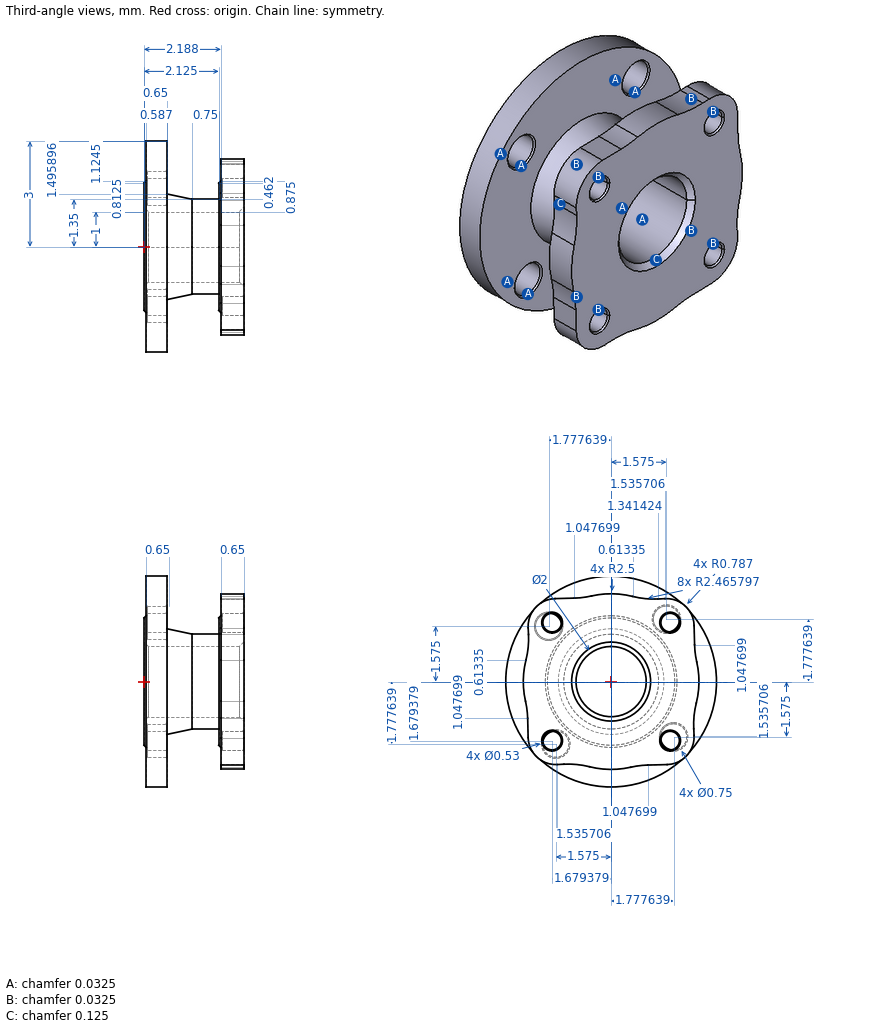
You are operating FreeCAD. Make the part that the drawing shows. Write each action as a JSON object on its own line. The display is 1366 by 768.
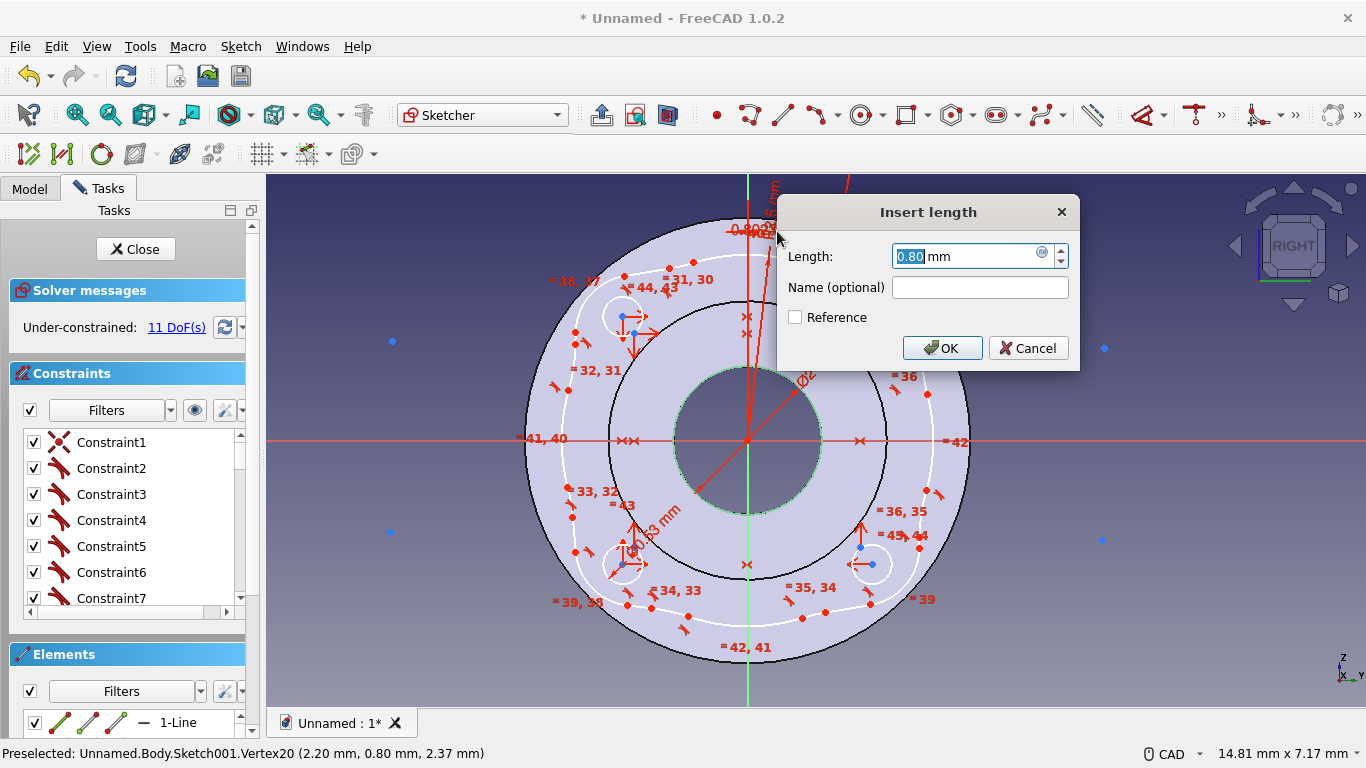
{"action": "type", "text": "0.61335"}
{"action": "key", "text": "Return"}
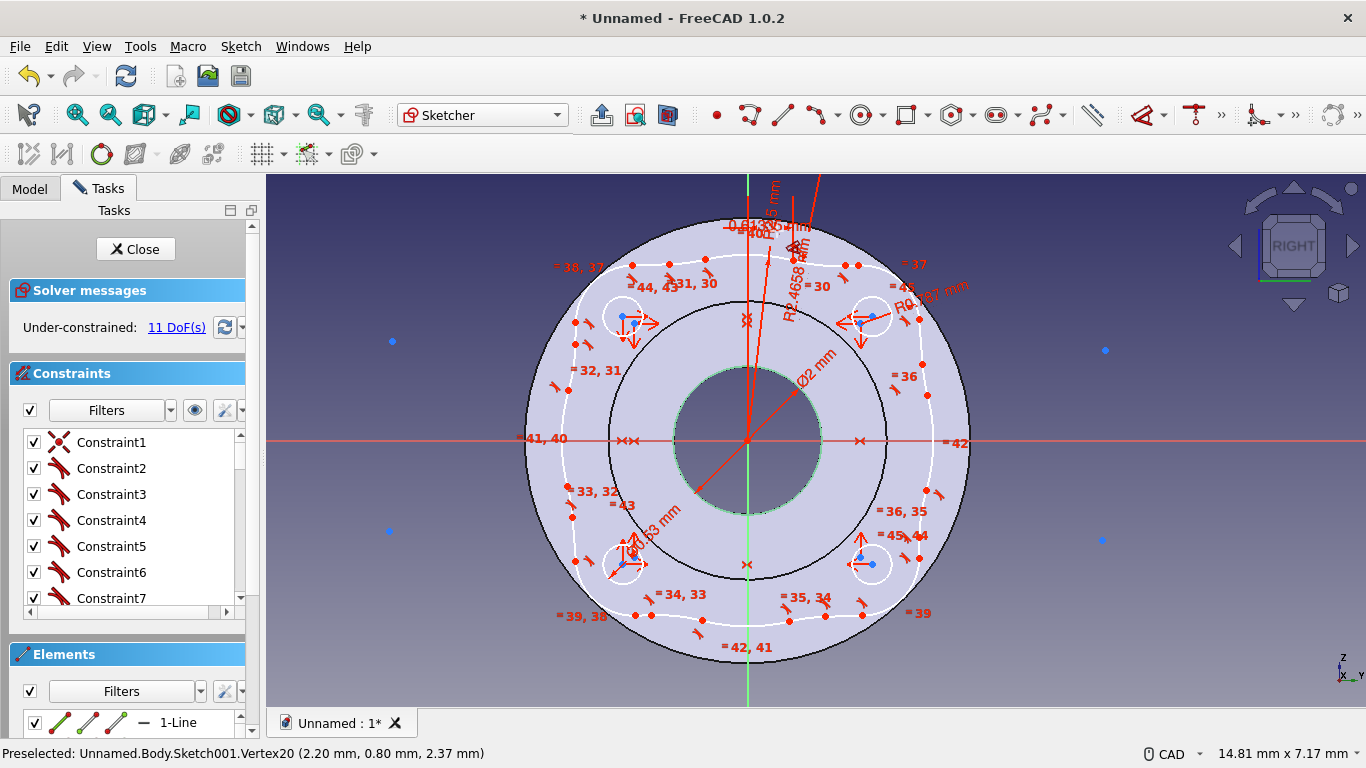
{"action": "left_click", "coordinate": [569, 391]}
{"action": "left_click", "coordinate": [535, 416]}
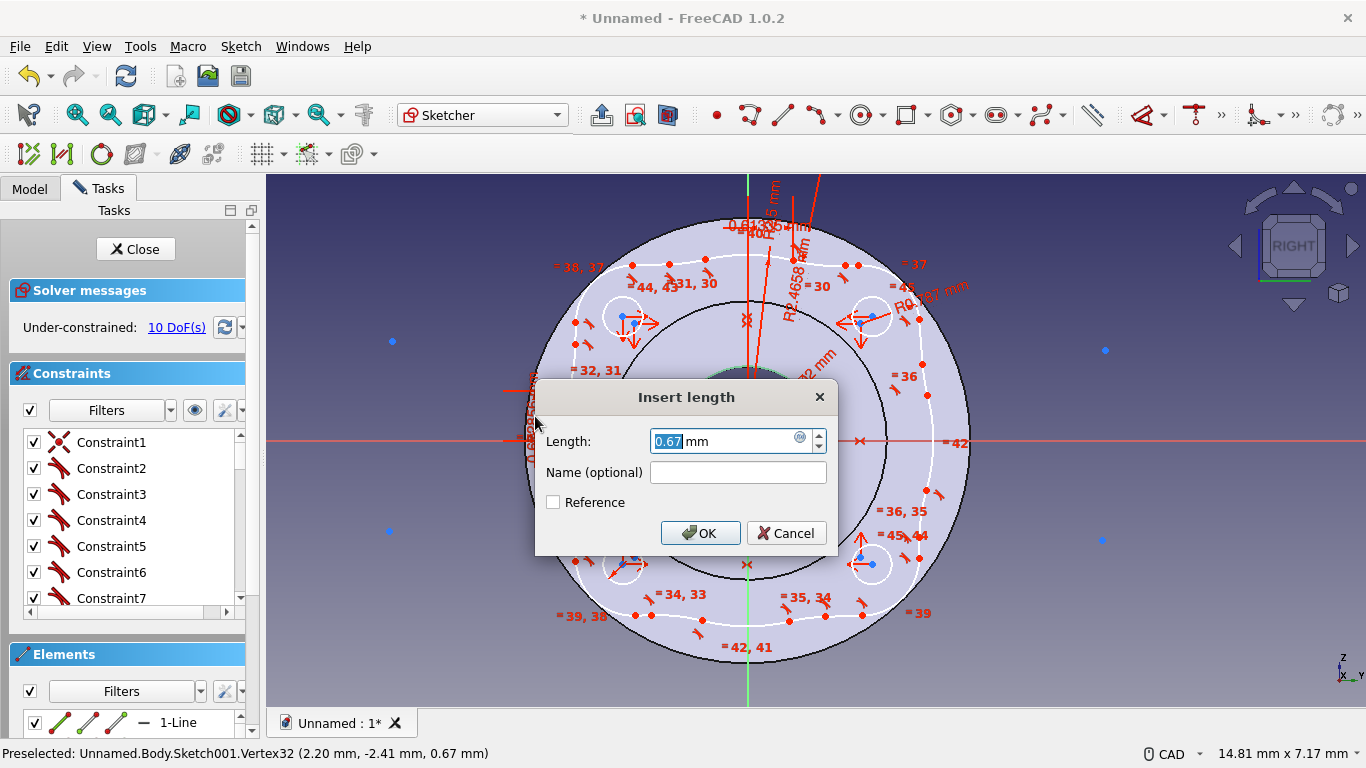
{"action": "type", "text": "0.61335"}
{"action": "key", "text": "Return"}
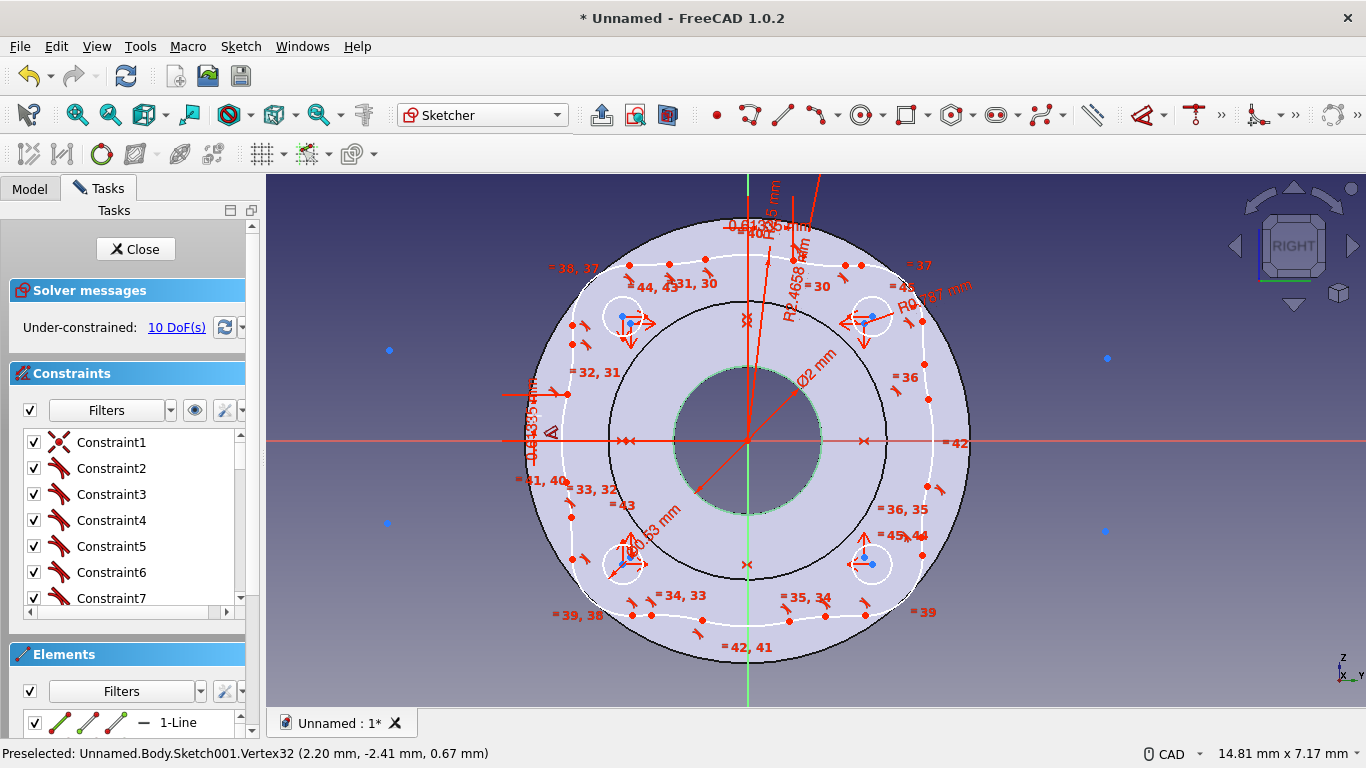
{"action": "left_click", "coordinate": [623, 564]}
{"action": "left_click", "coordinate": [685, 598]}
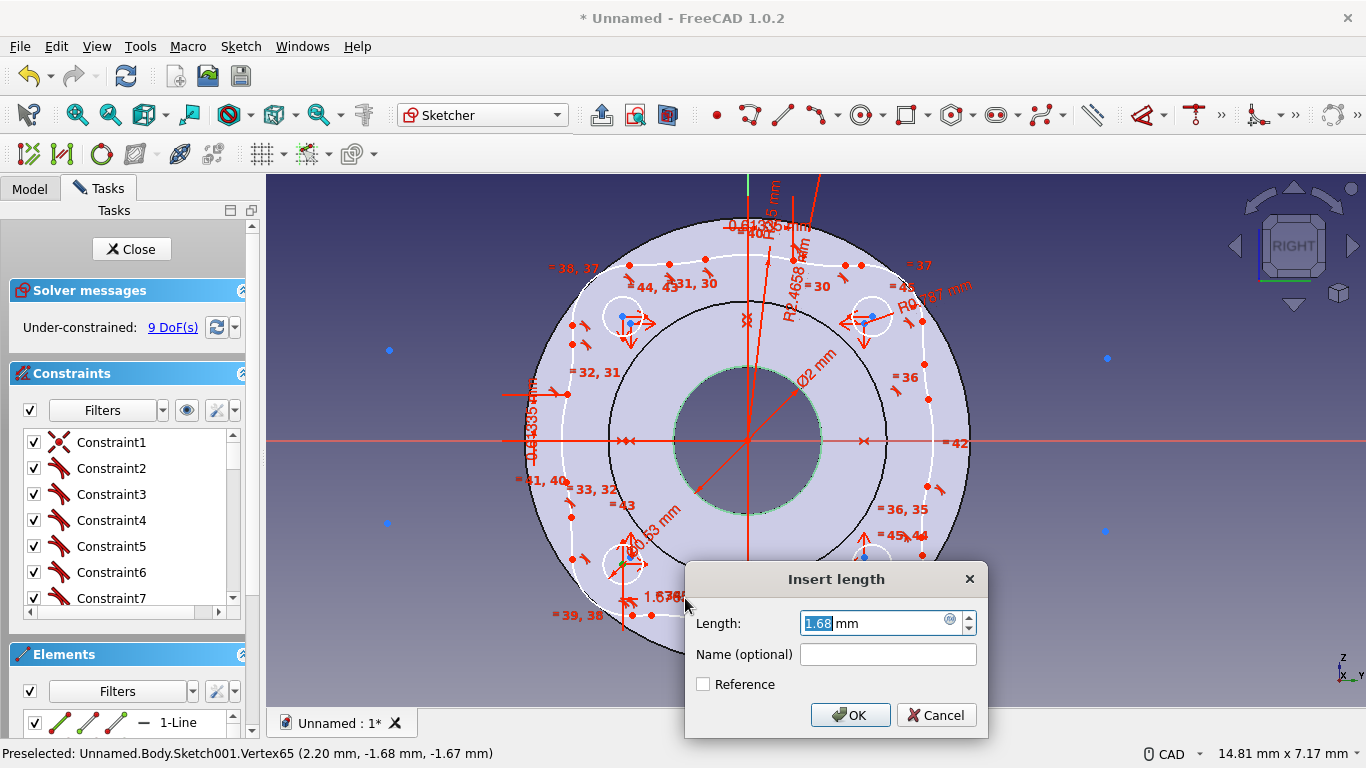
{"action": "type", "text": "1.679379"}
{"action": "key", "text": "Return"}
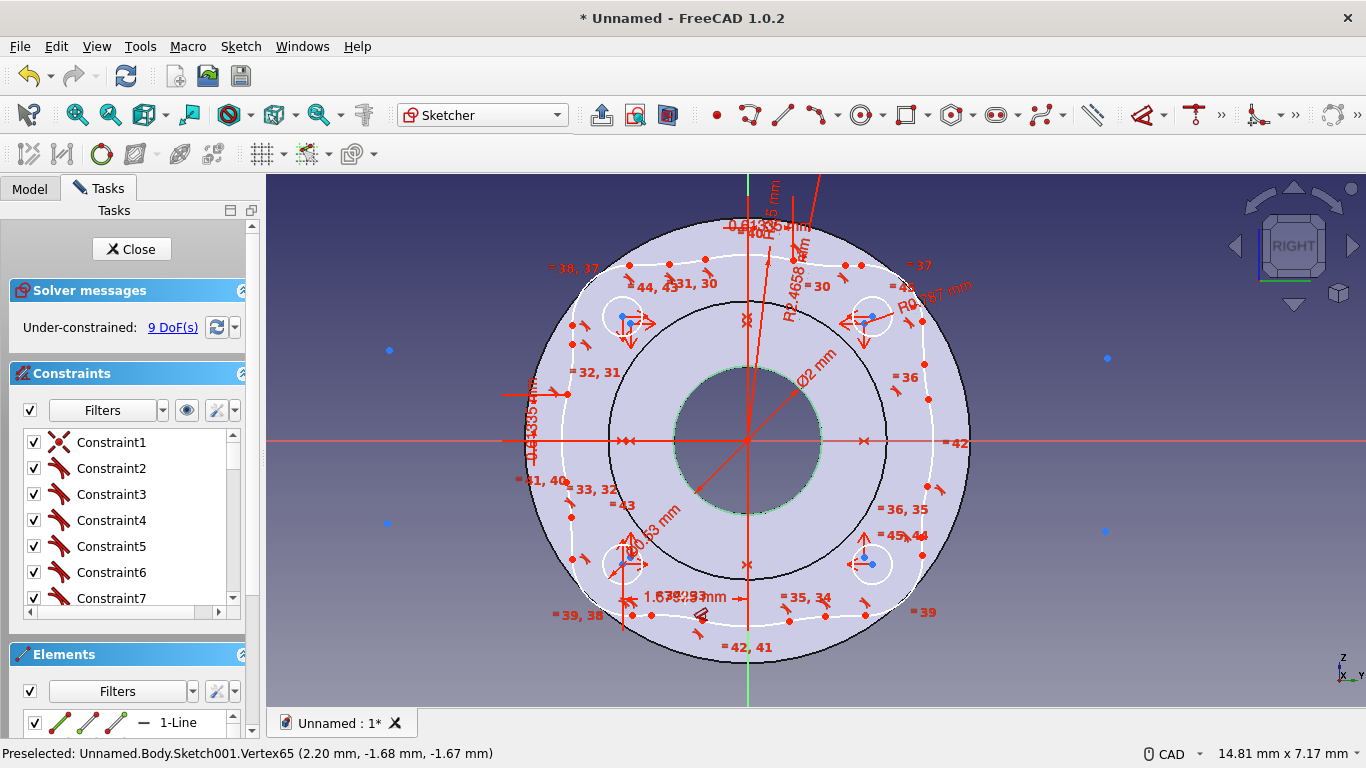
{"action": "left_click", "coordinate": [623, 564]}
{"action": "left_click", "coordinate": [589, 503]}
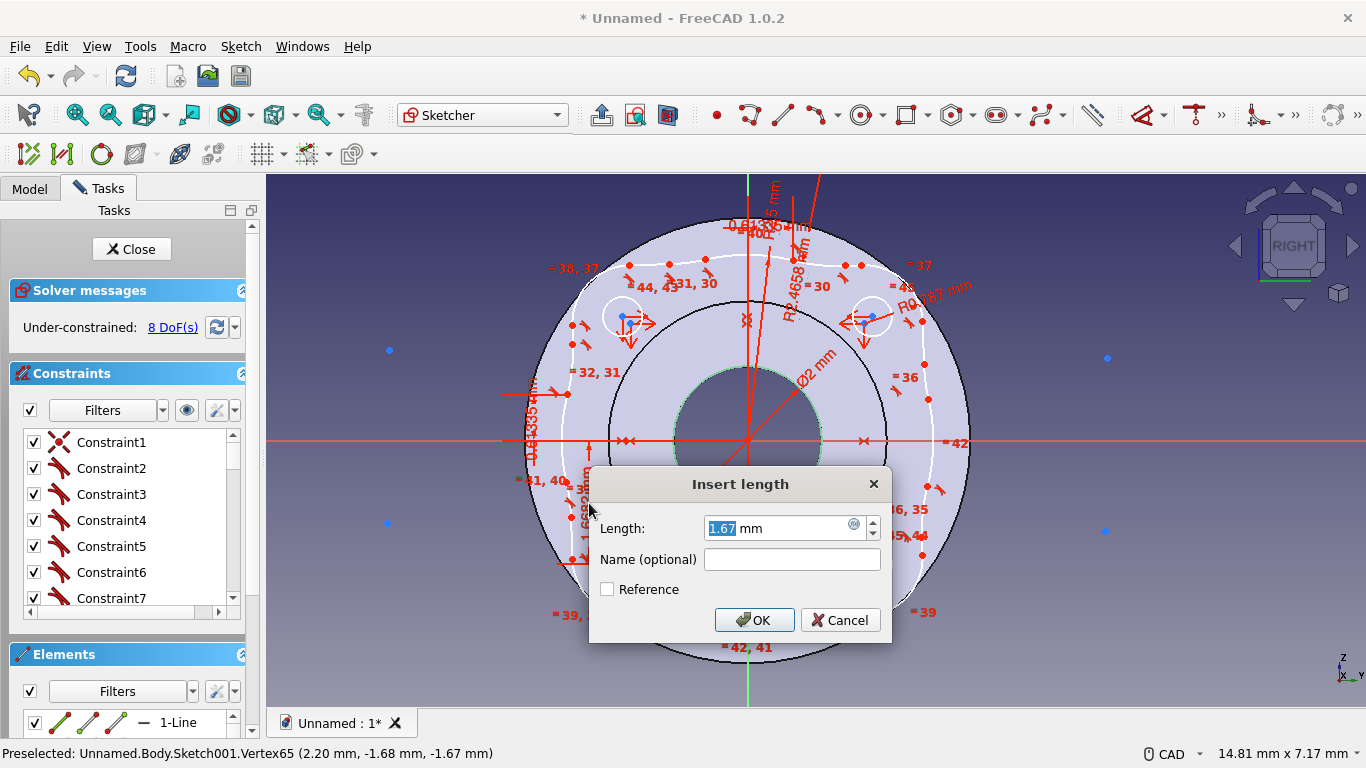
{"action": "type", "text": "1.679379"}
{"action": "key", "text": "Return"}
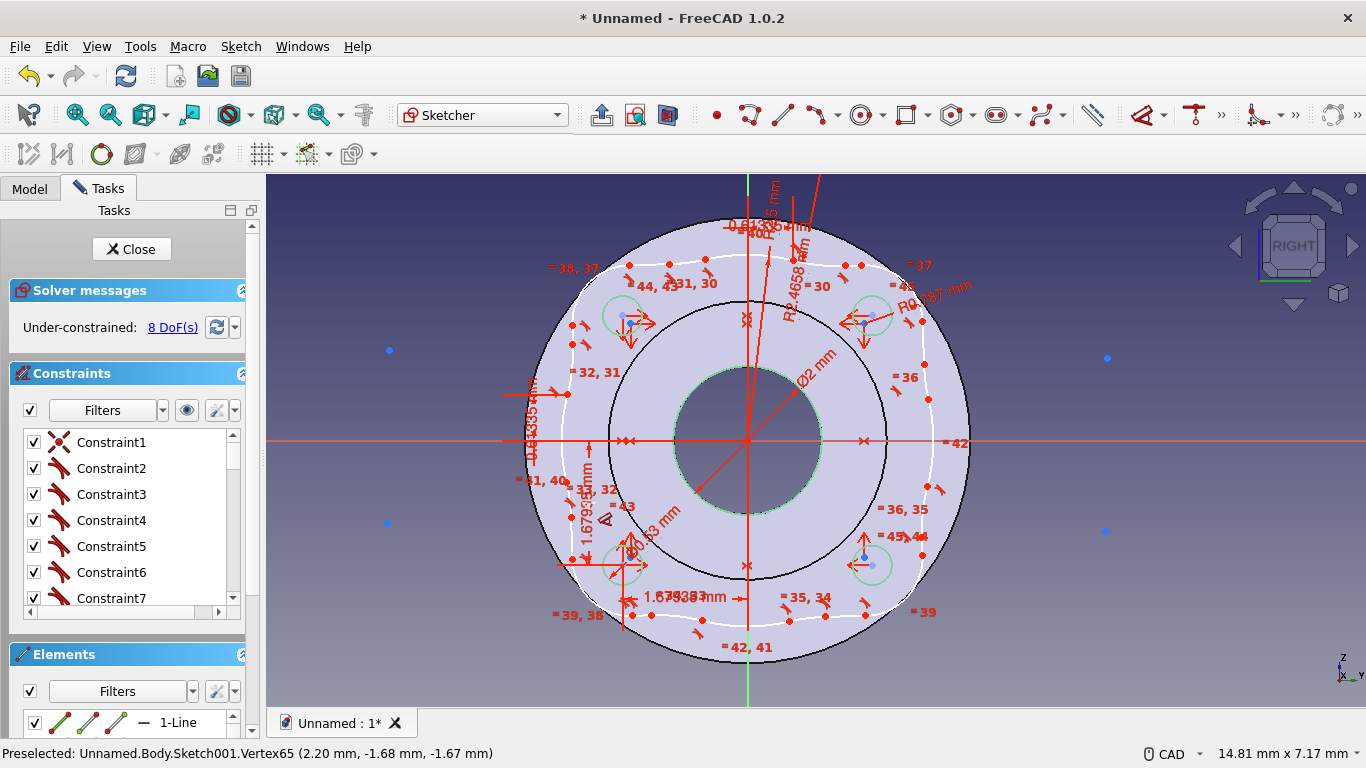
{"action": "left_click", "coordinate": [924, 365]}
{"action": "left_click", "coordinate": [958, 403]}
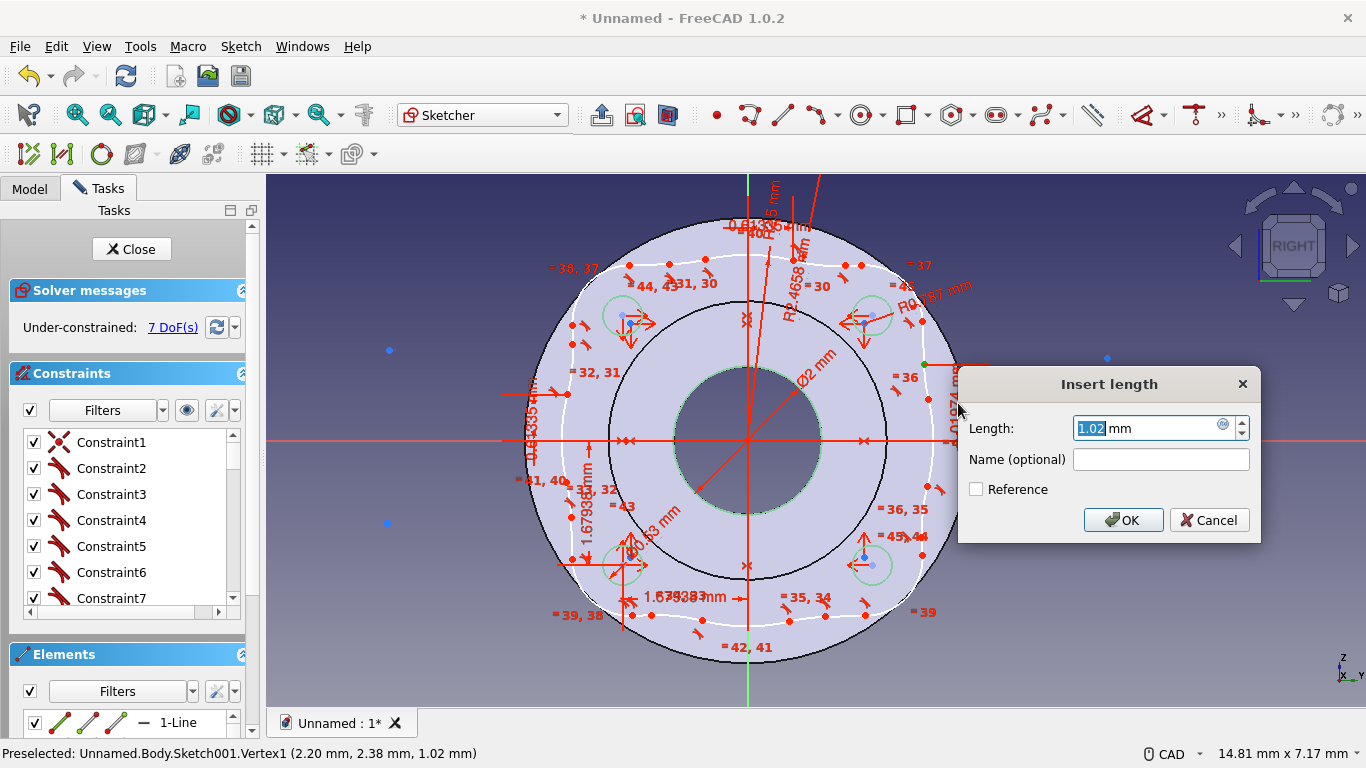
{"action": "type", "text": "1.047699"}
{"action": "key", "text": "Return"}